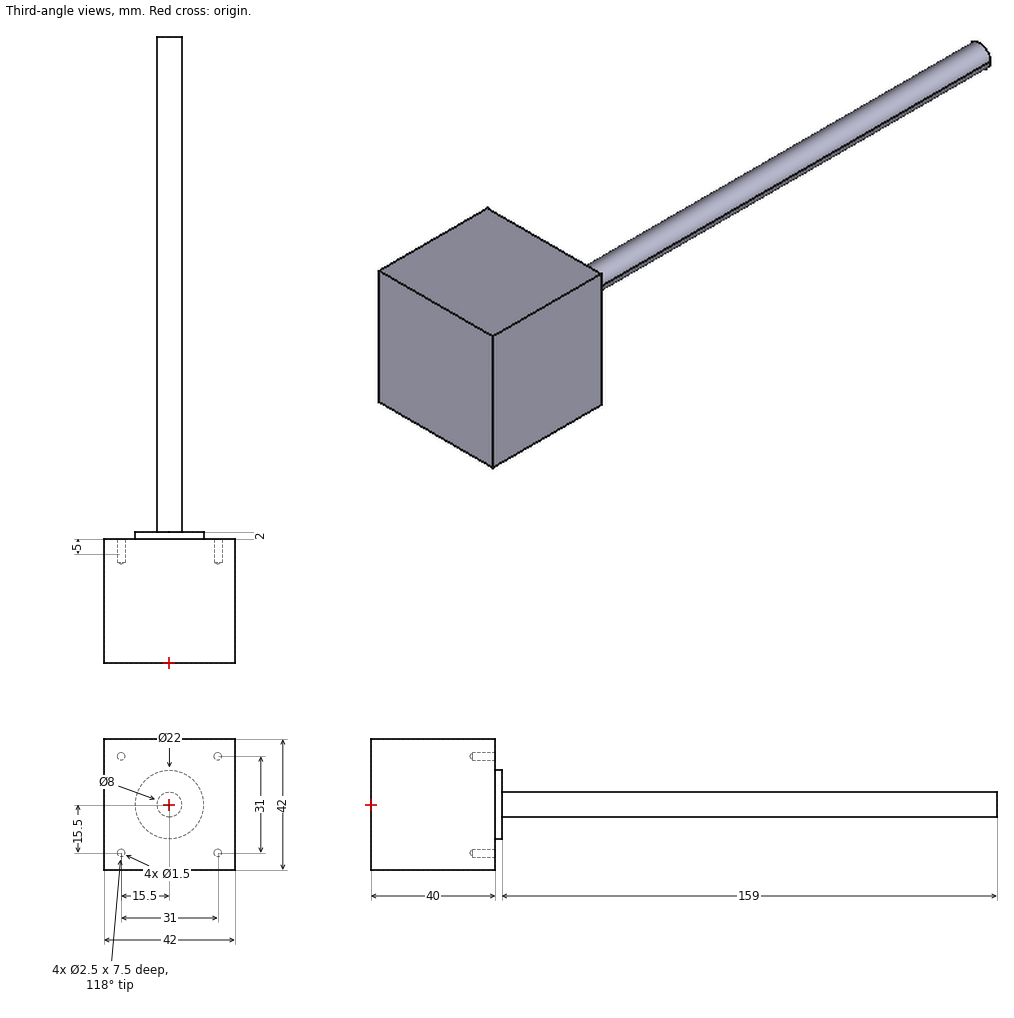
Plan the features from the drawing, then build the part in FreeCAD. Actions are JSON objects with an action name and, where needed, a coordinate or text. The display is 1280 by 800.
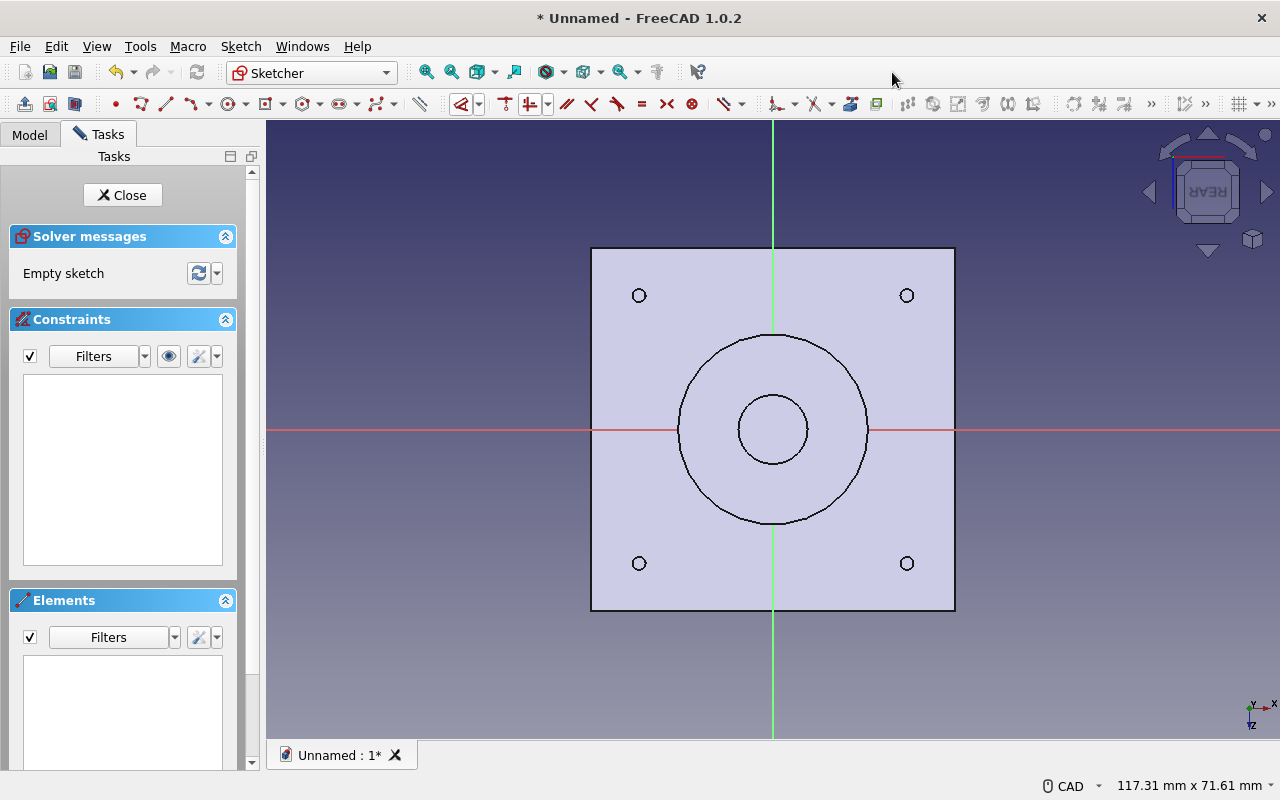
{"action": "key", "text": "q s"}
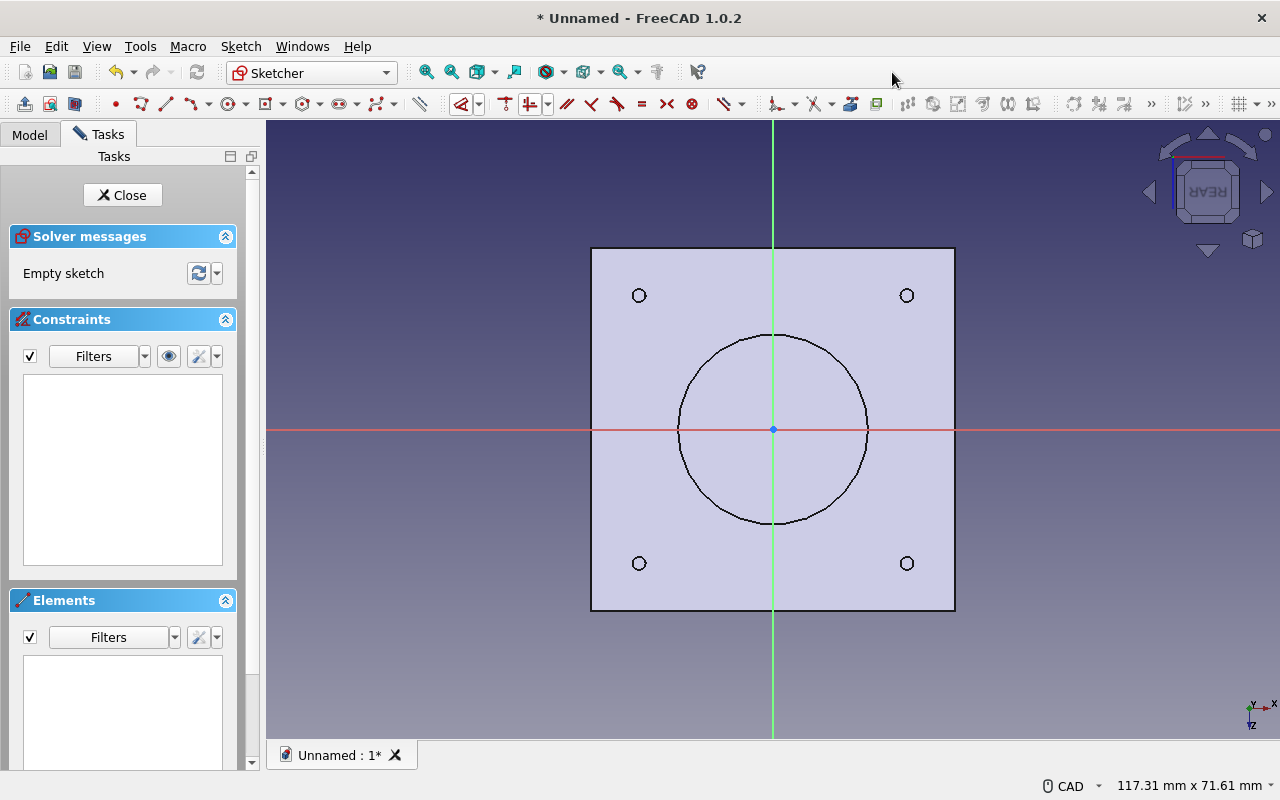
{"action": "scroll", "coordinate": [912, 429], "scroll_direction": "up", "scroll_amount": 2}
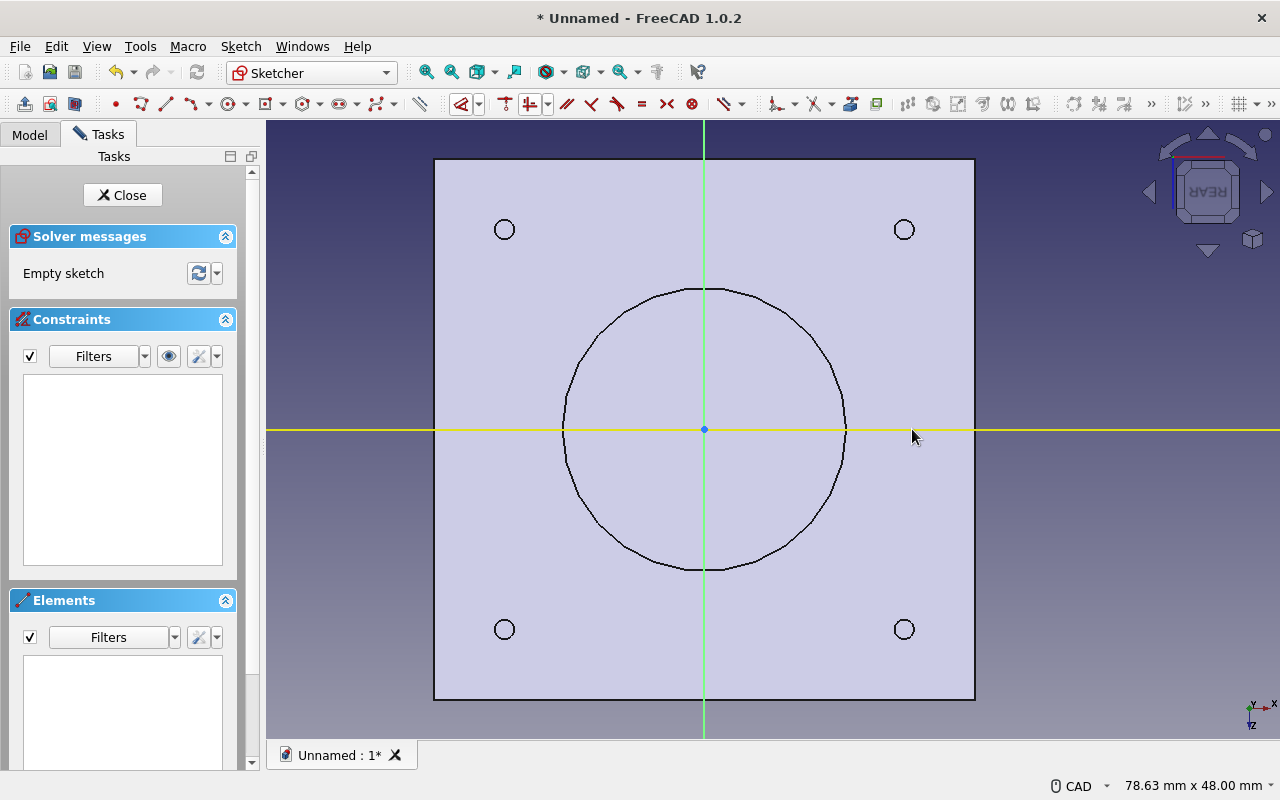
{"action": "key", "text": "g c"}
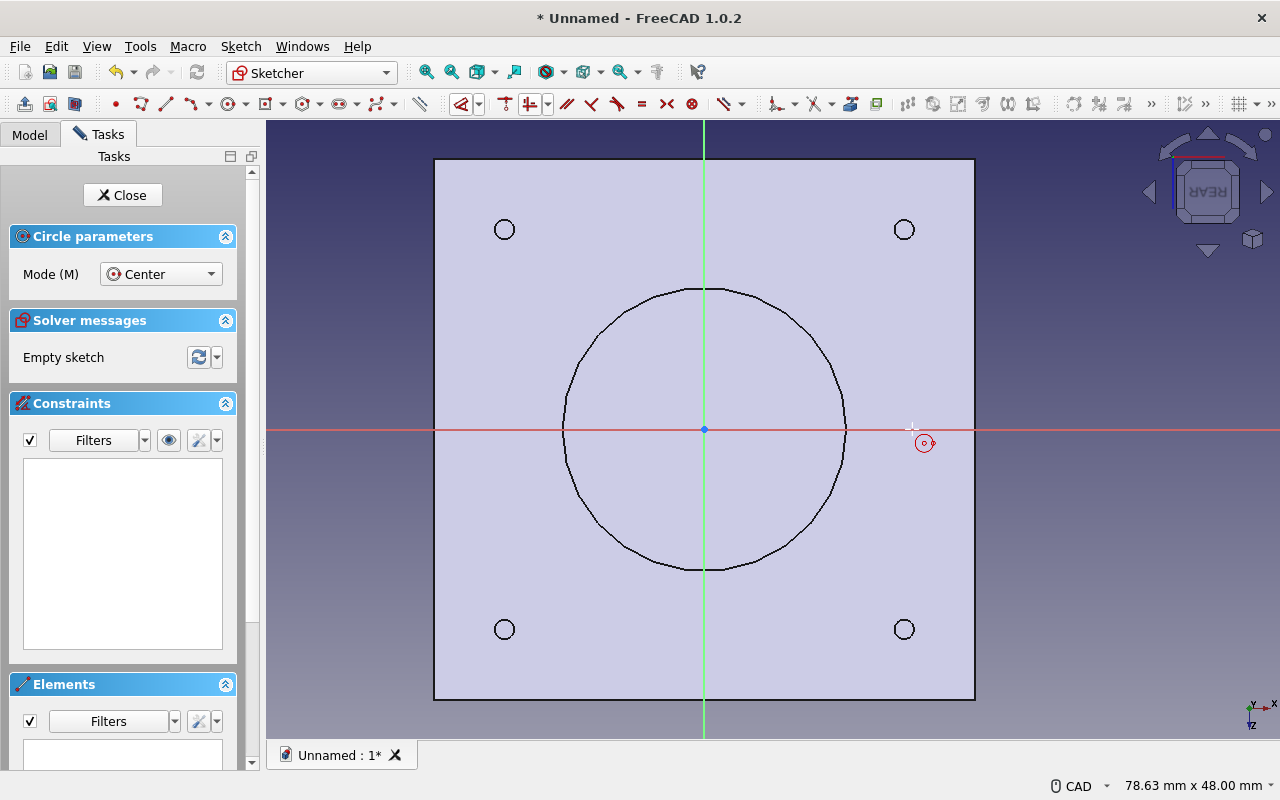
{"action": "scroll", "coordinate": [504, 230], "scroll_direction": "up", "scroll_amount": 2}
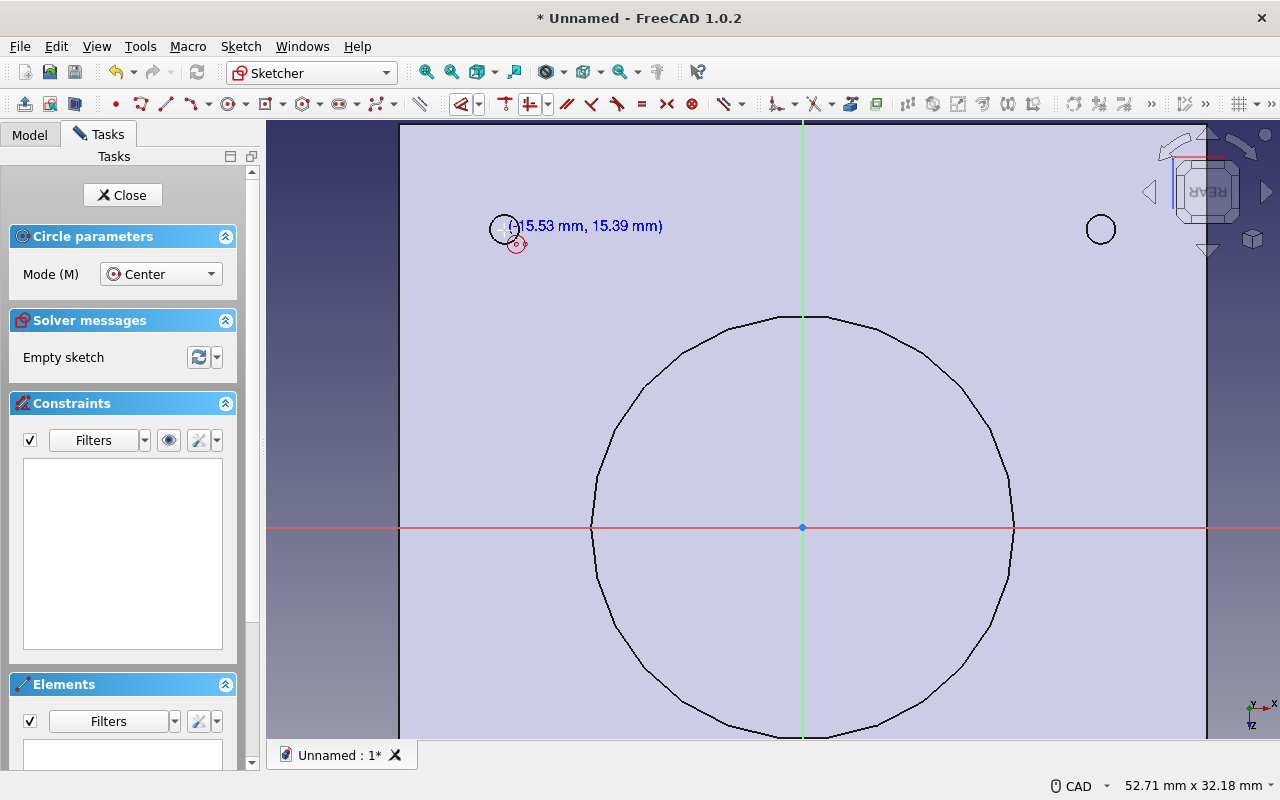
{"action": "left_click", "coordinate": [505, 229]}
{"action": "left_click", "coordinate": [522, 212]}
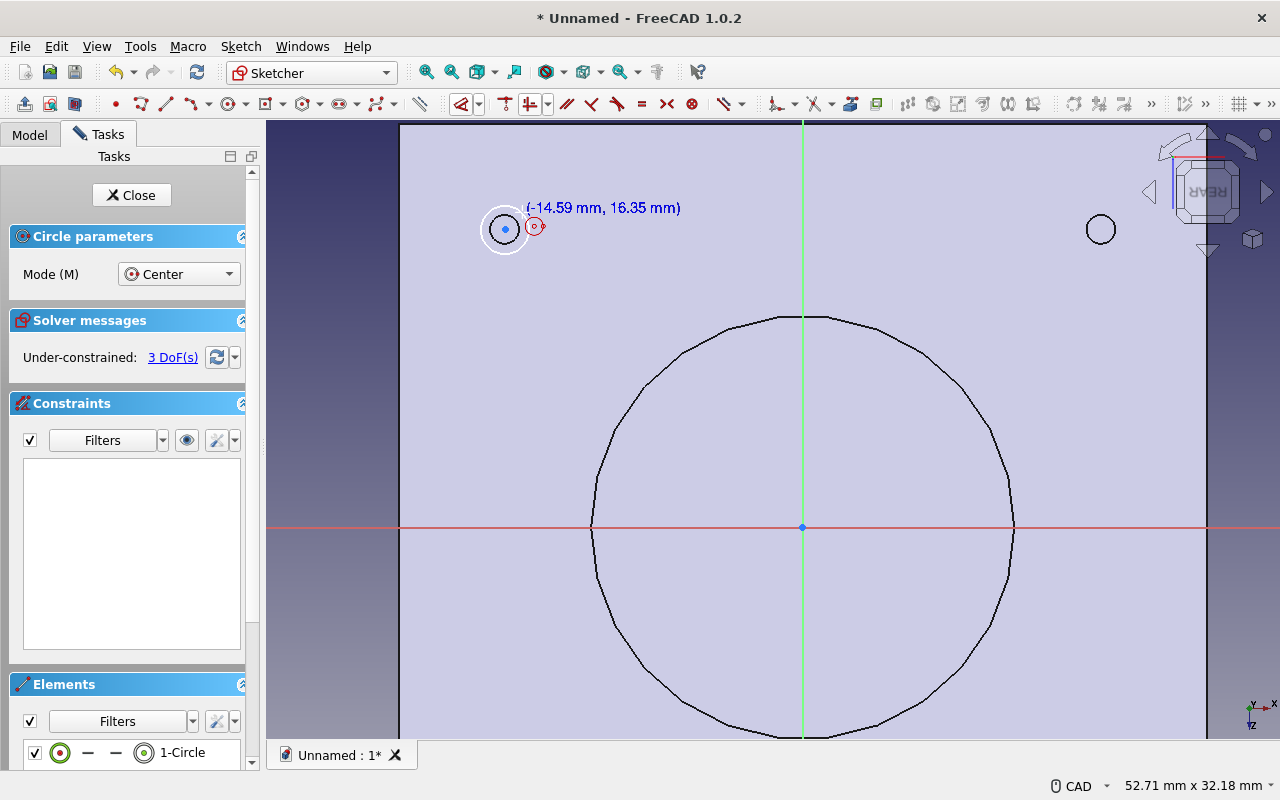
{"action": "scroll", "coordinate": [505, 230], "scroll_direction": "down", "scroll_amount": 2}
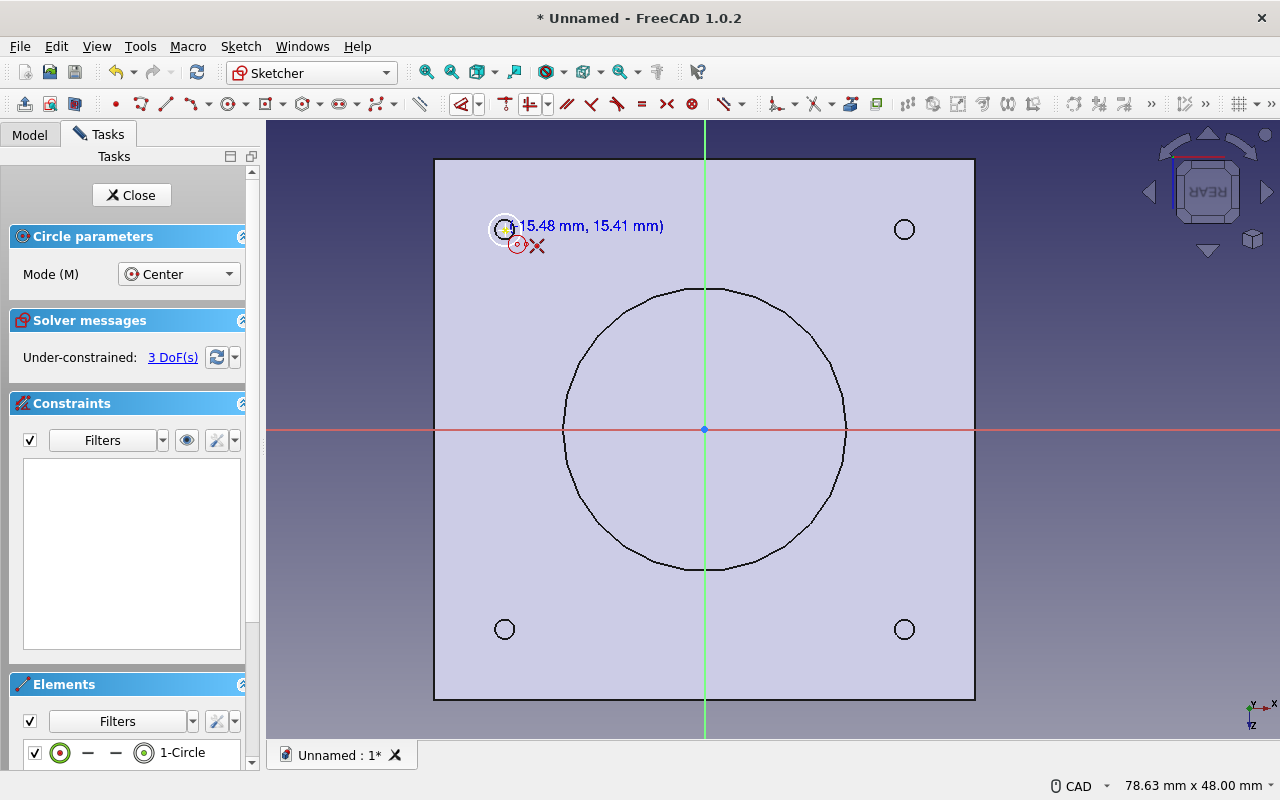
{"action": "scroll", "coordinate": [905, 629], "scroll_direction": "up", "scroll_amount": 2}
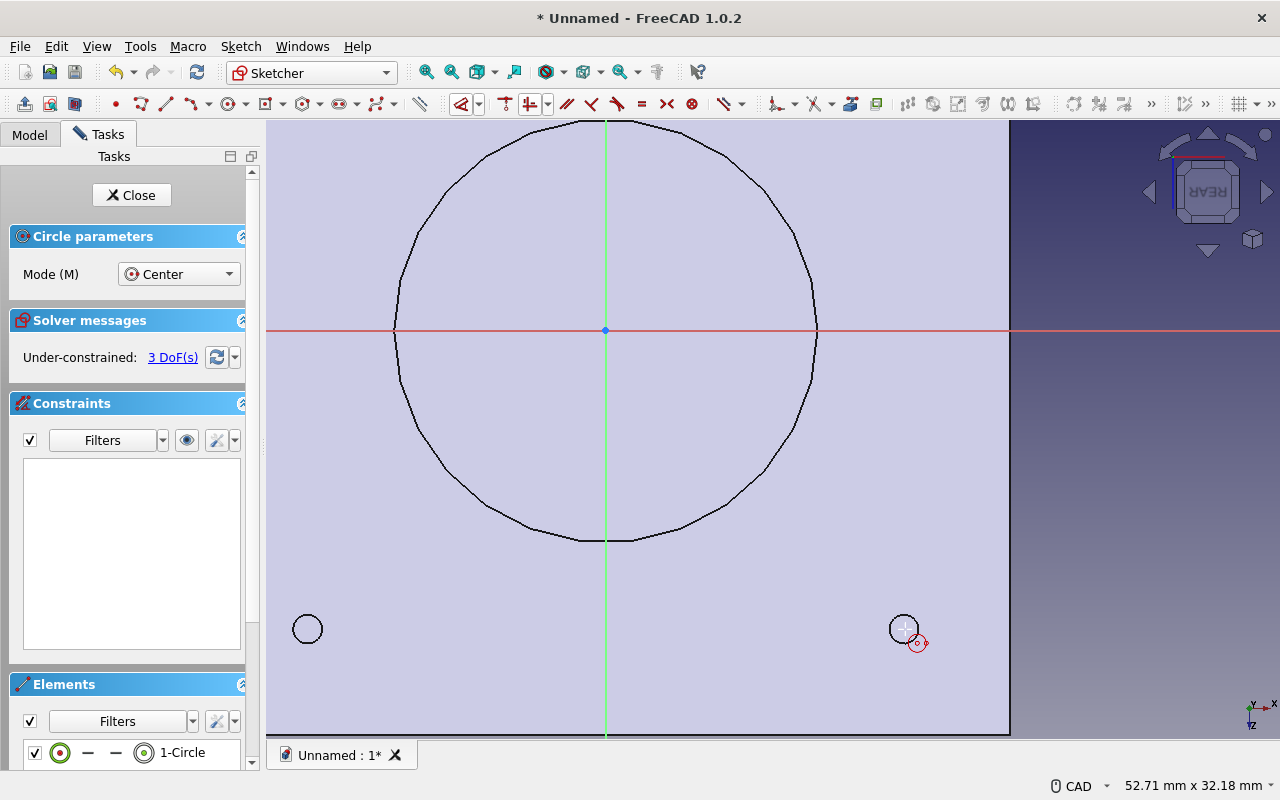
{"action": "left_click", "coordinate": [904, 629]}
{"action": "left_click", "coordinate": [921, 612]}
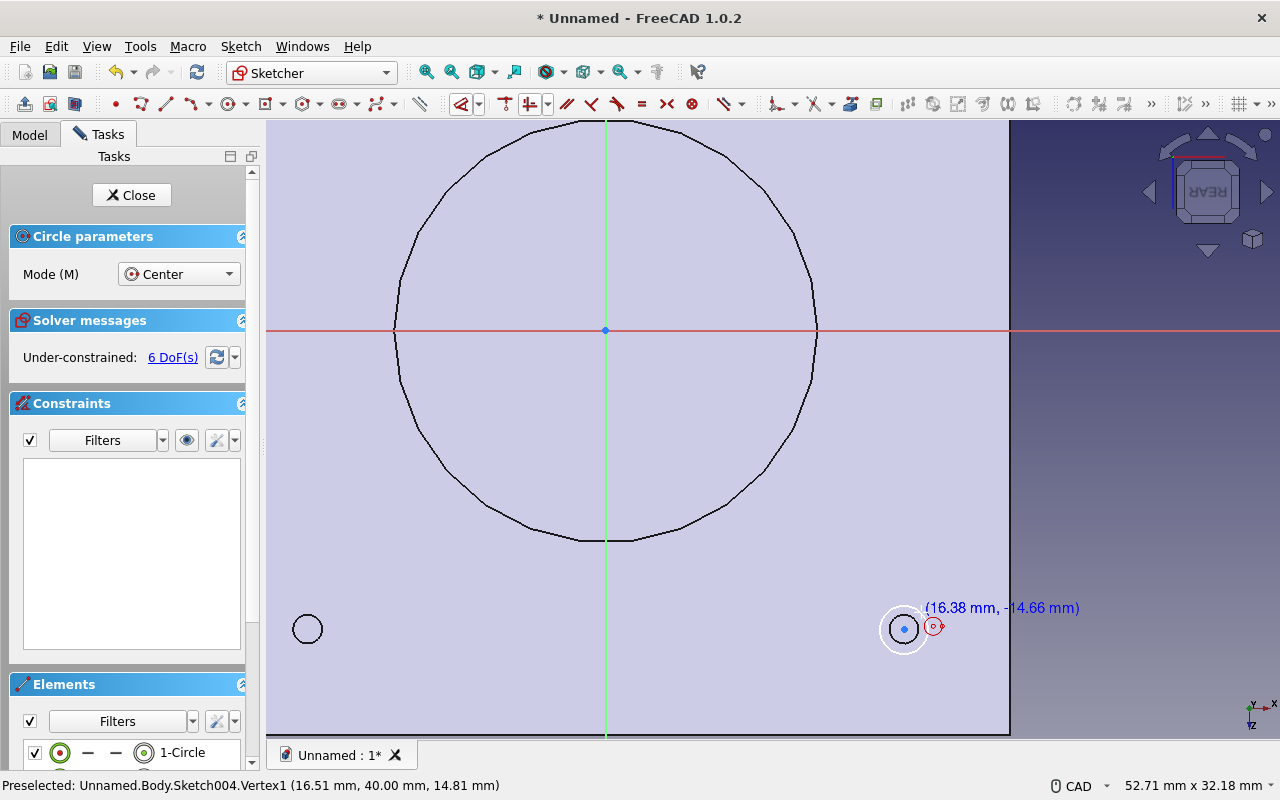
{"action": "left_click", "coordinate": [308, 629]}
{"action": "left_click", "coordinate": [325, 612]}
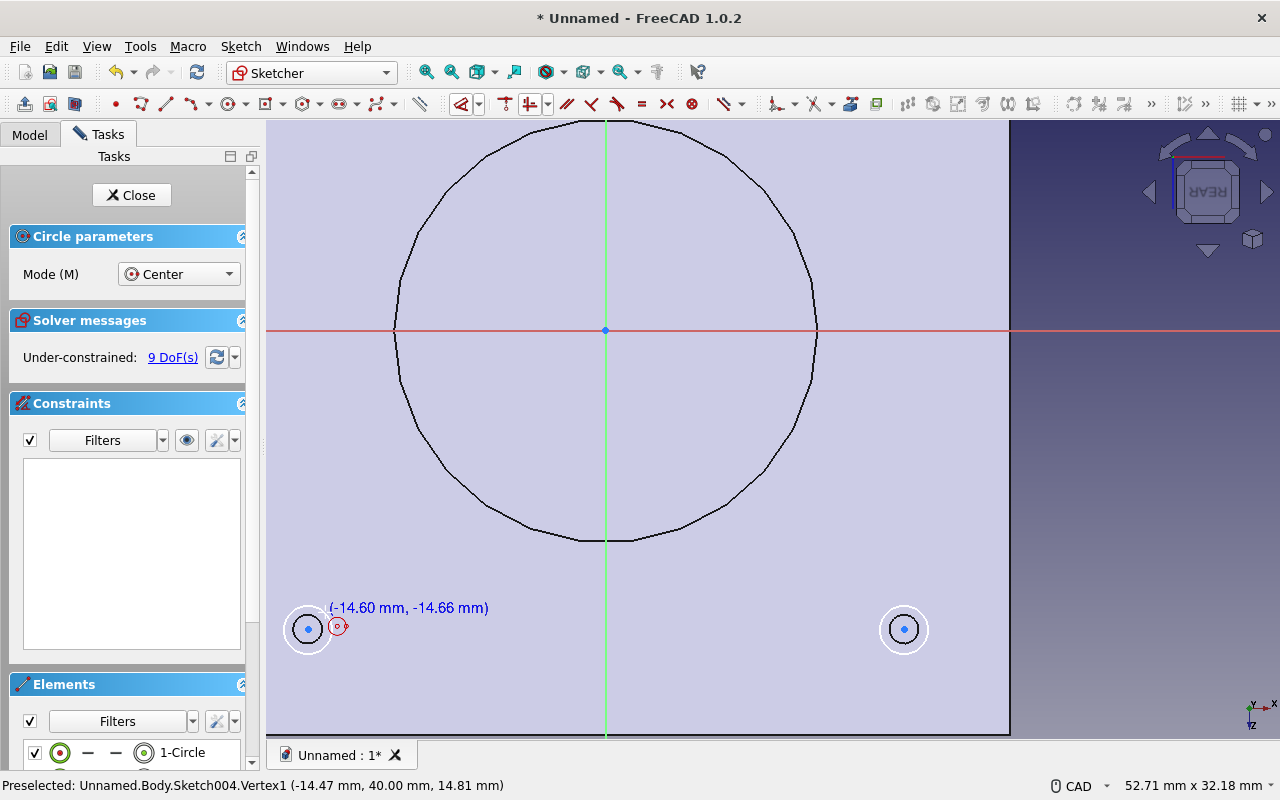
{"action": "scroll", "coordinate": [905, 630], "scroll_direction": "down", "scroll_amount": 2}